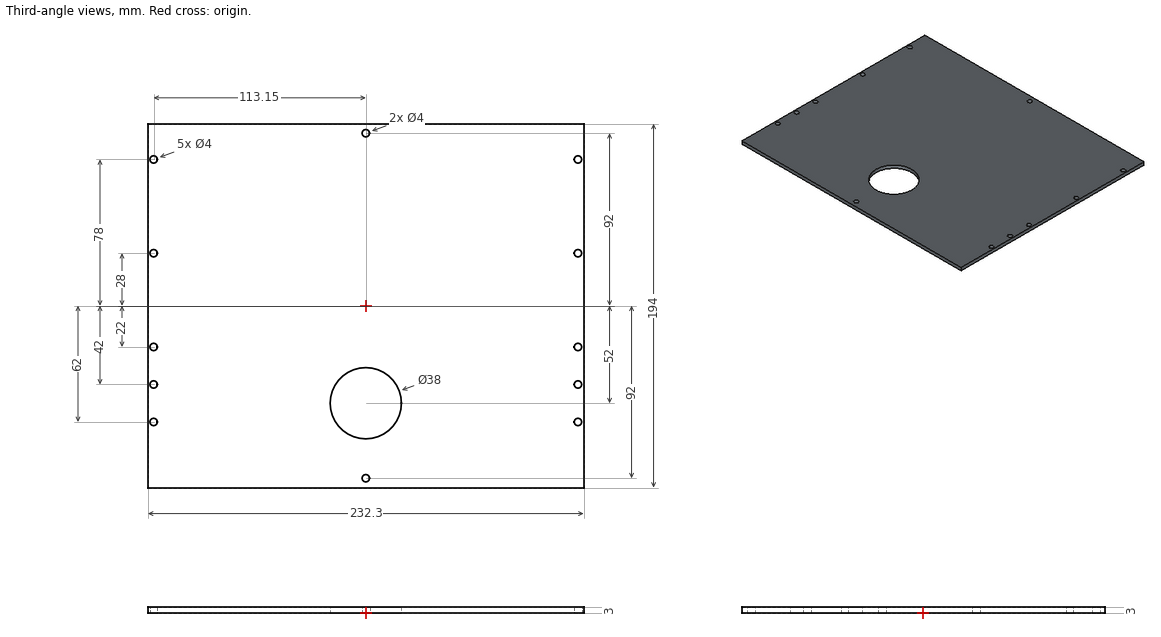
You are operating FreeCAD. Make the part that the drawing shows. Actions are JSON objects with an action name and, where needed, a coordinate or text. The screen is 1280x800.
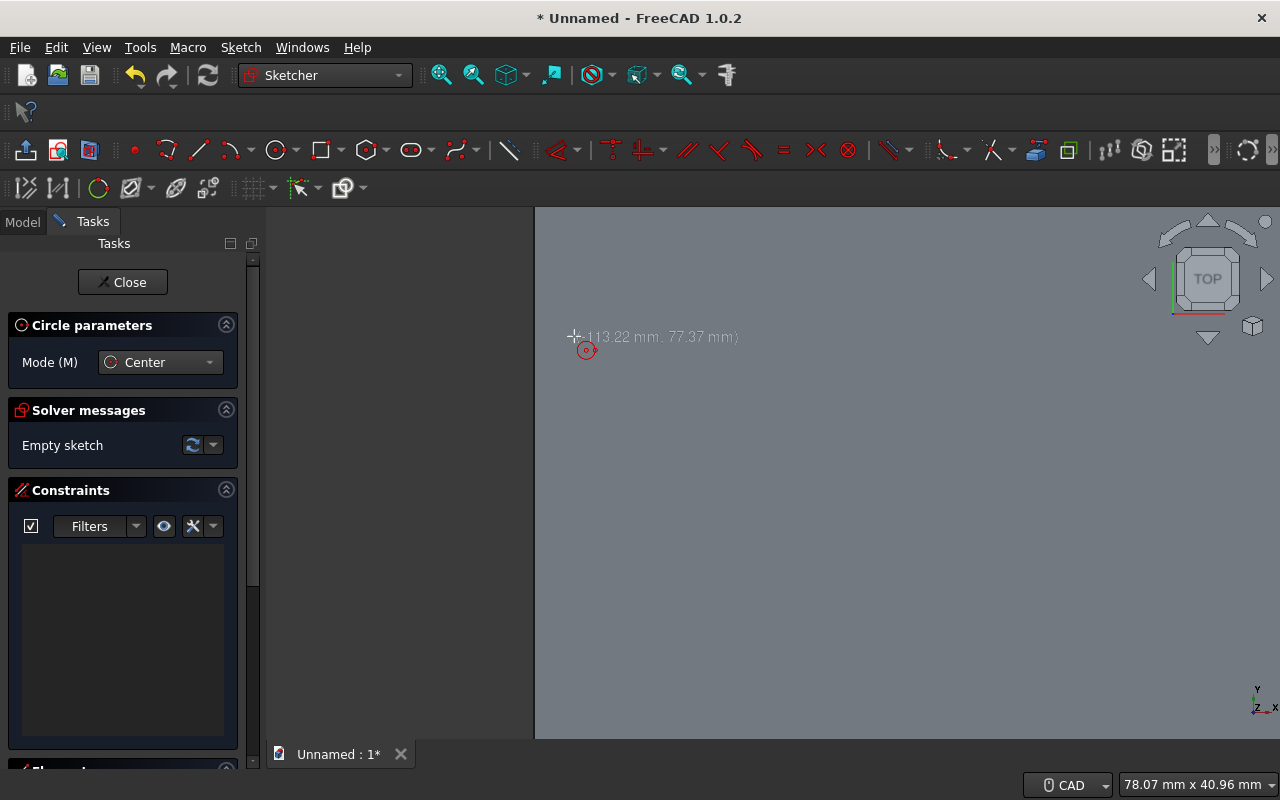
{"action": "scroll", "coordinate": [588, 321], "scroll_direction": "down", "scroll_amount": 9}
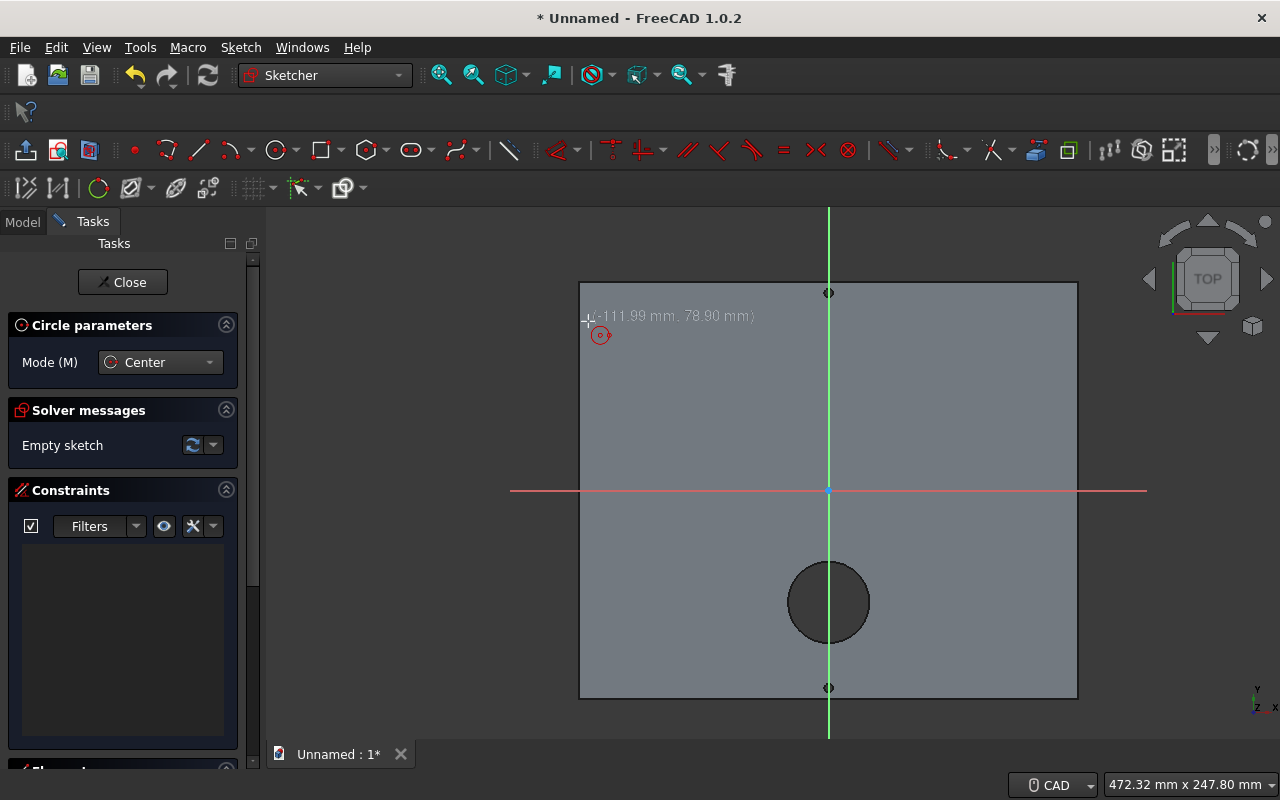
{"action": "left_click", "coordinate": [586, 323]}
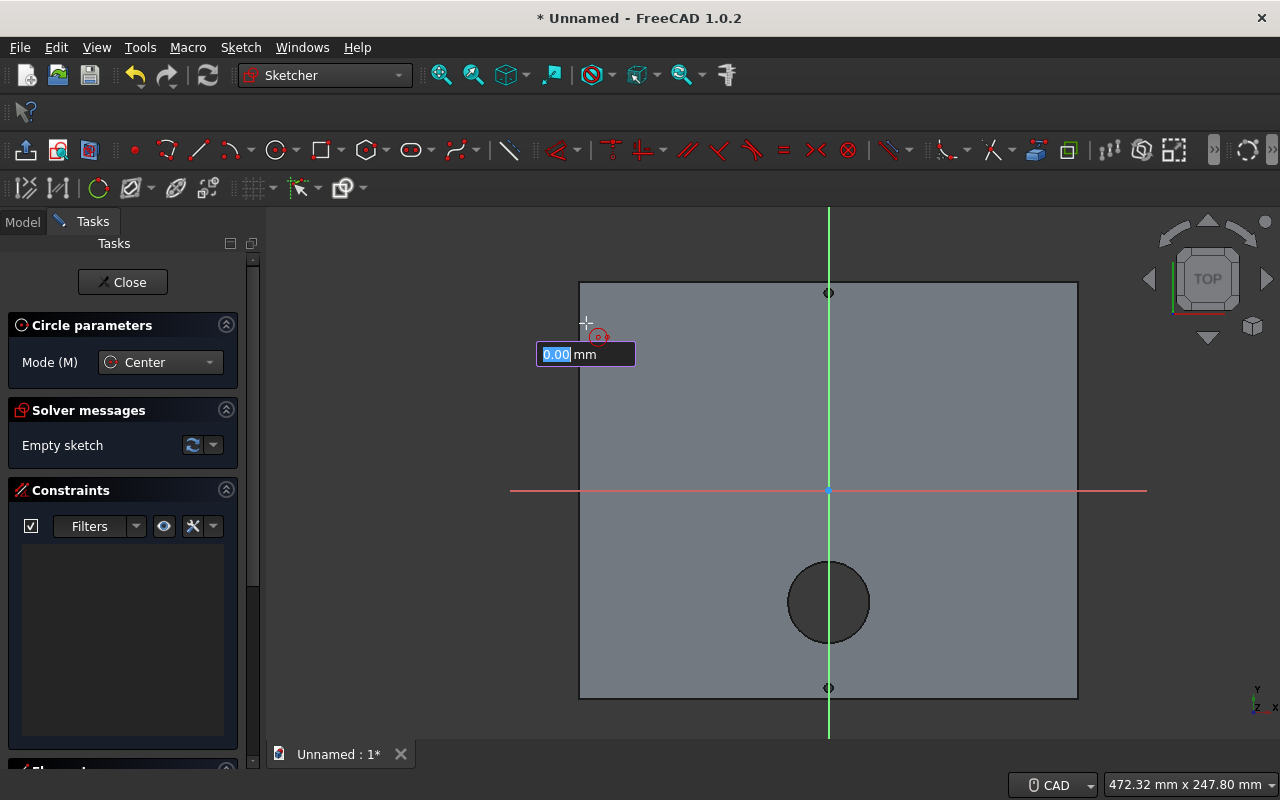
{"action": "scroll", "coordinate": [589, 320], "scroll_direction": "up", "scroll_amount": 7}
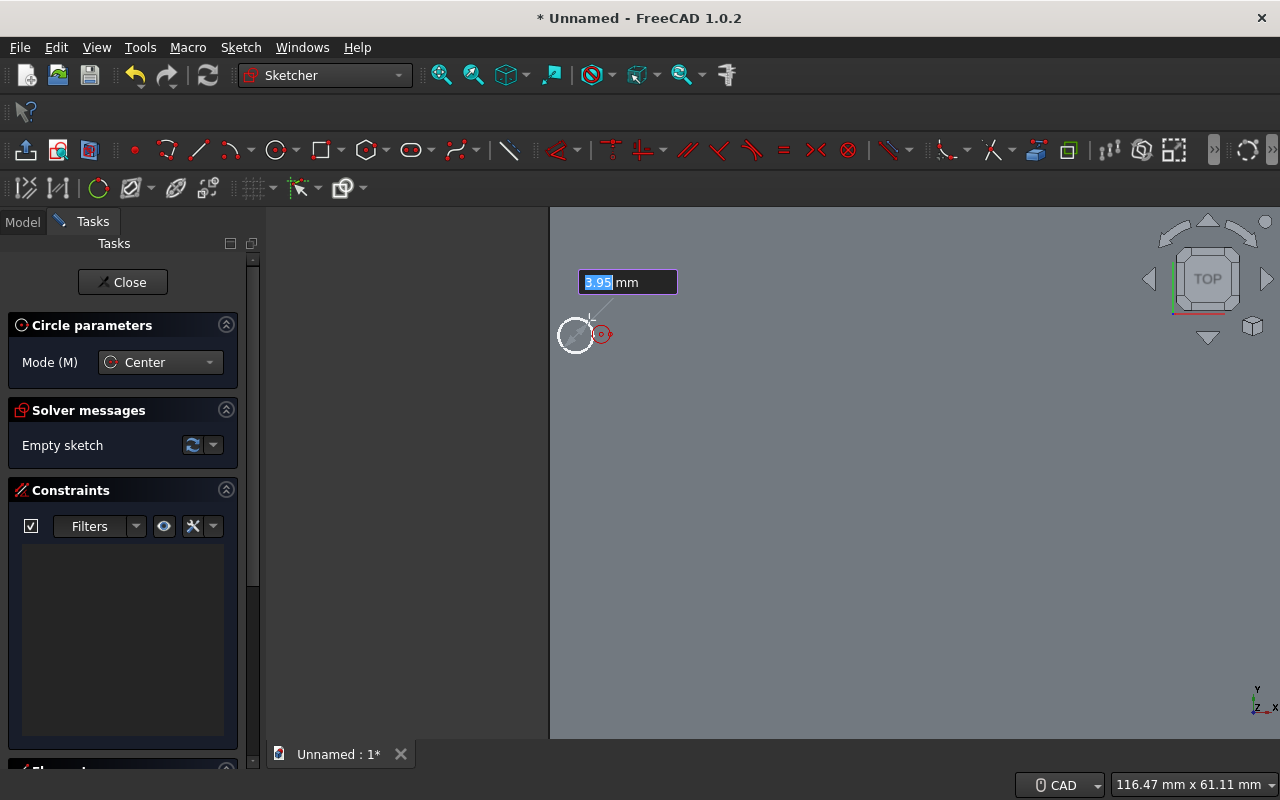
{"action": "left_click", "coordinate": [587, 320]}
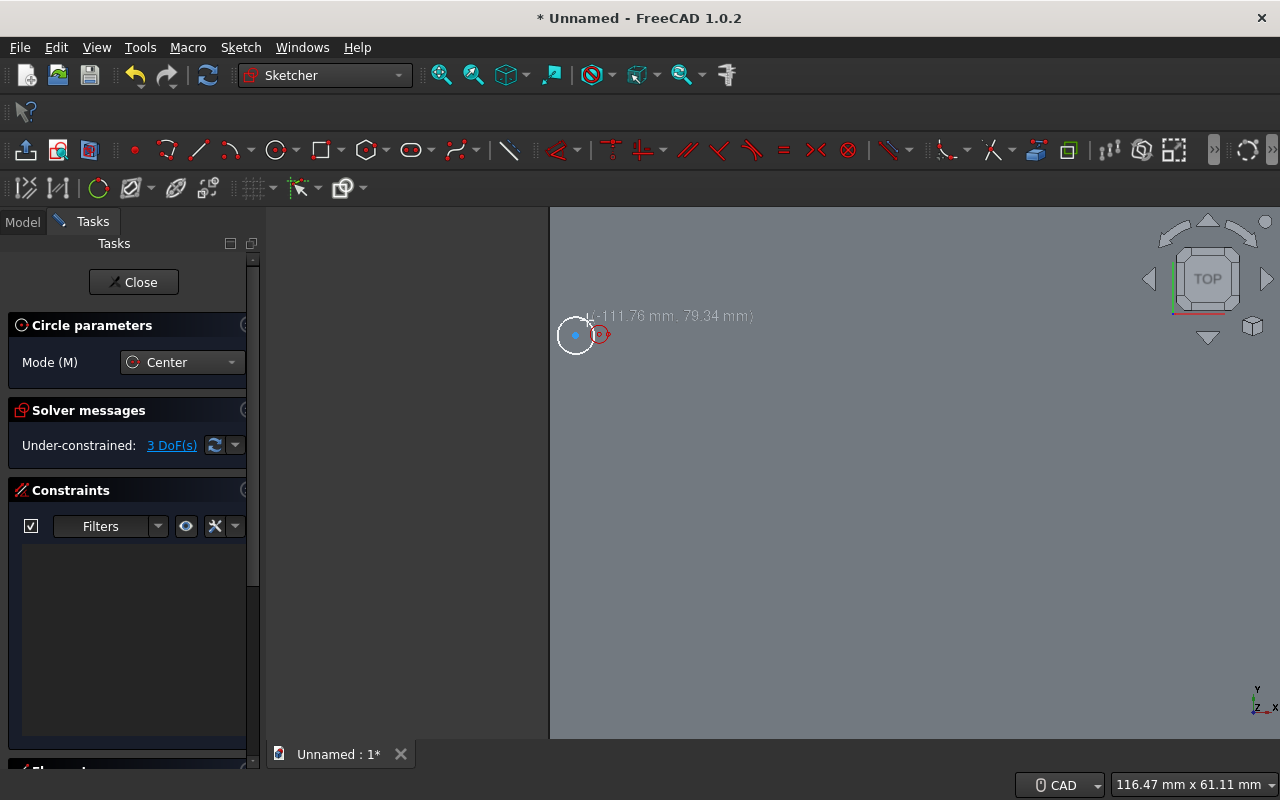
{"action": "scroll", "coordinate": [589, 319], "scroll_direction": "down", "scroll_amount": 7}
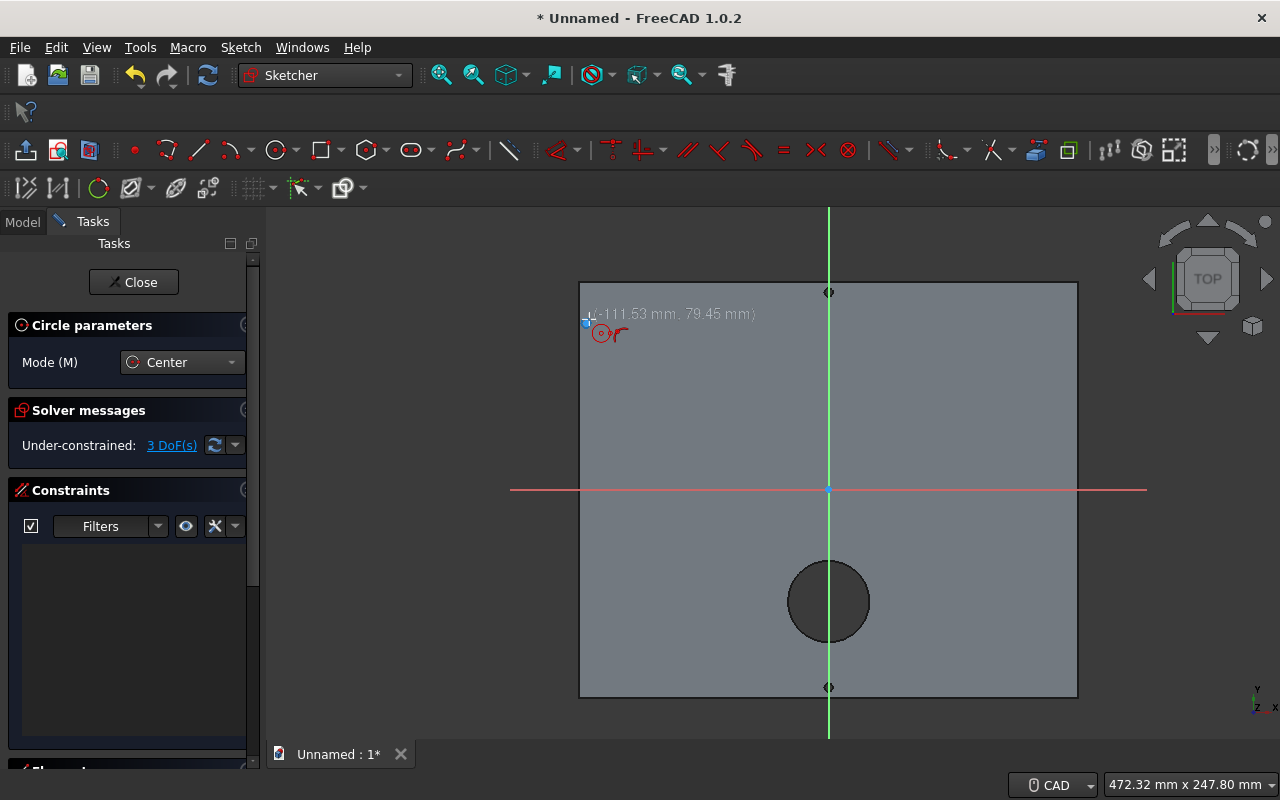
{"action": "scroll", "coordinate": [586, 430], "scroll_direction": "up", "scroll_amount": 9}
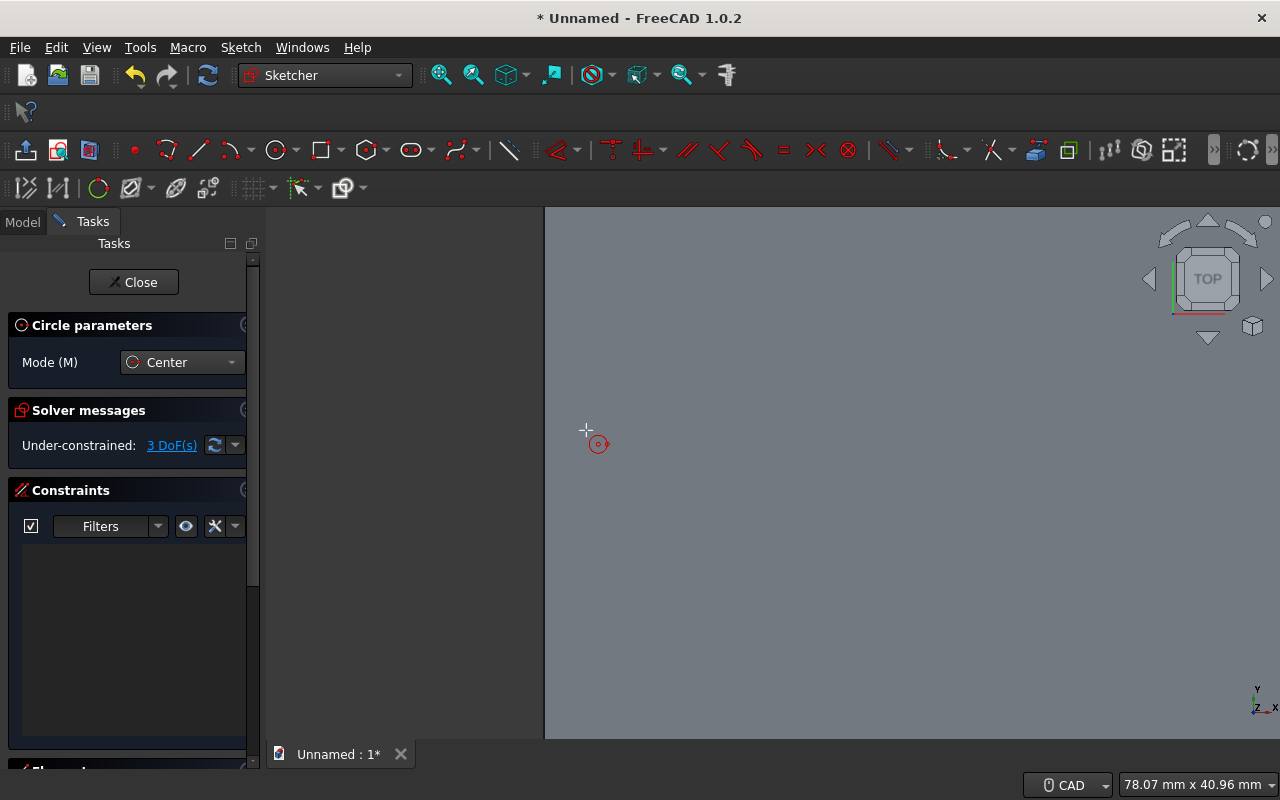
{"action": "scroll", "coordinate": [586, 431], "scroll_direction": "down", "scroll_amount": 9}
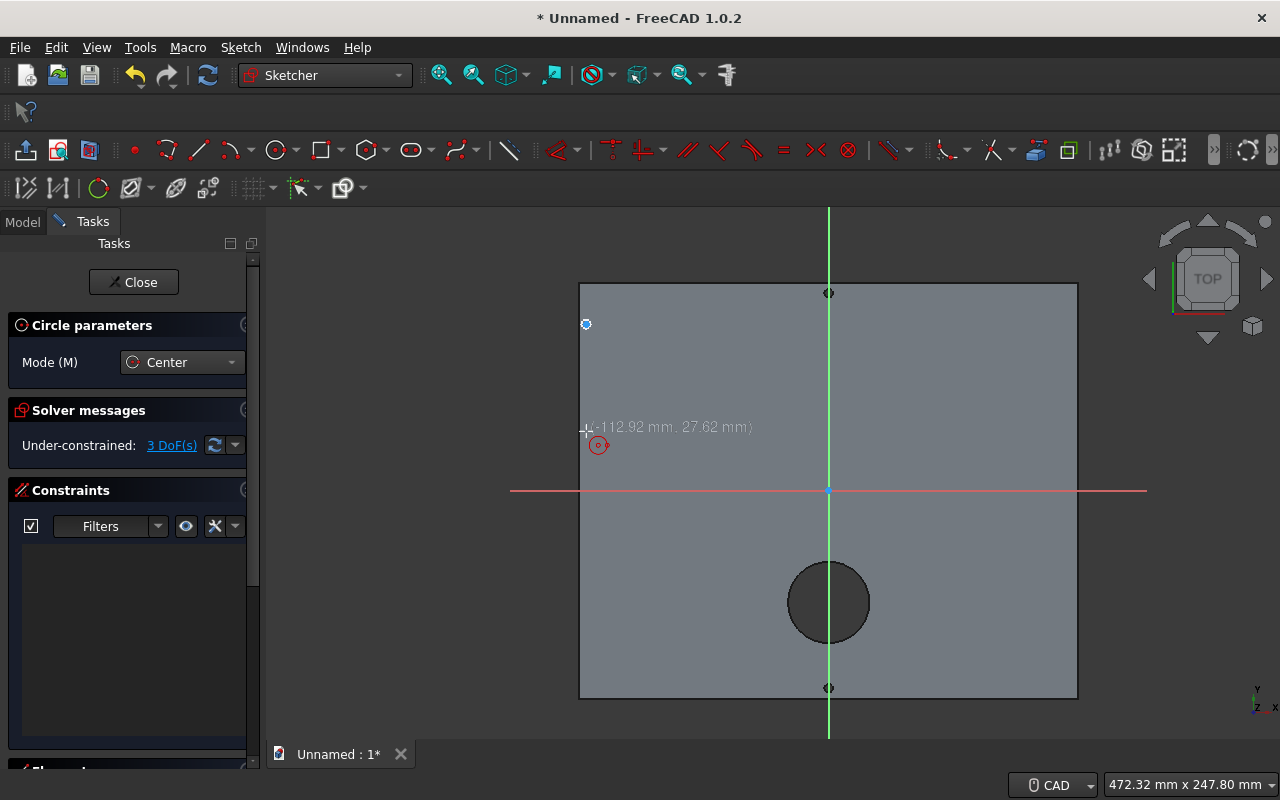
{"action": "left_click", "coordinate": [586, 431]}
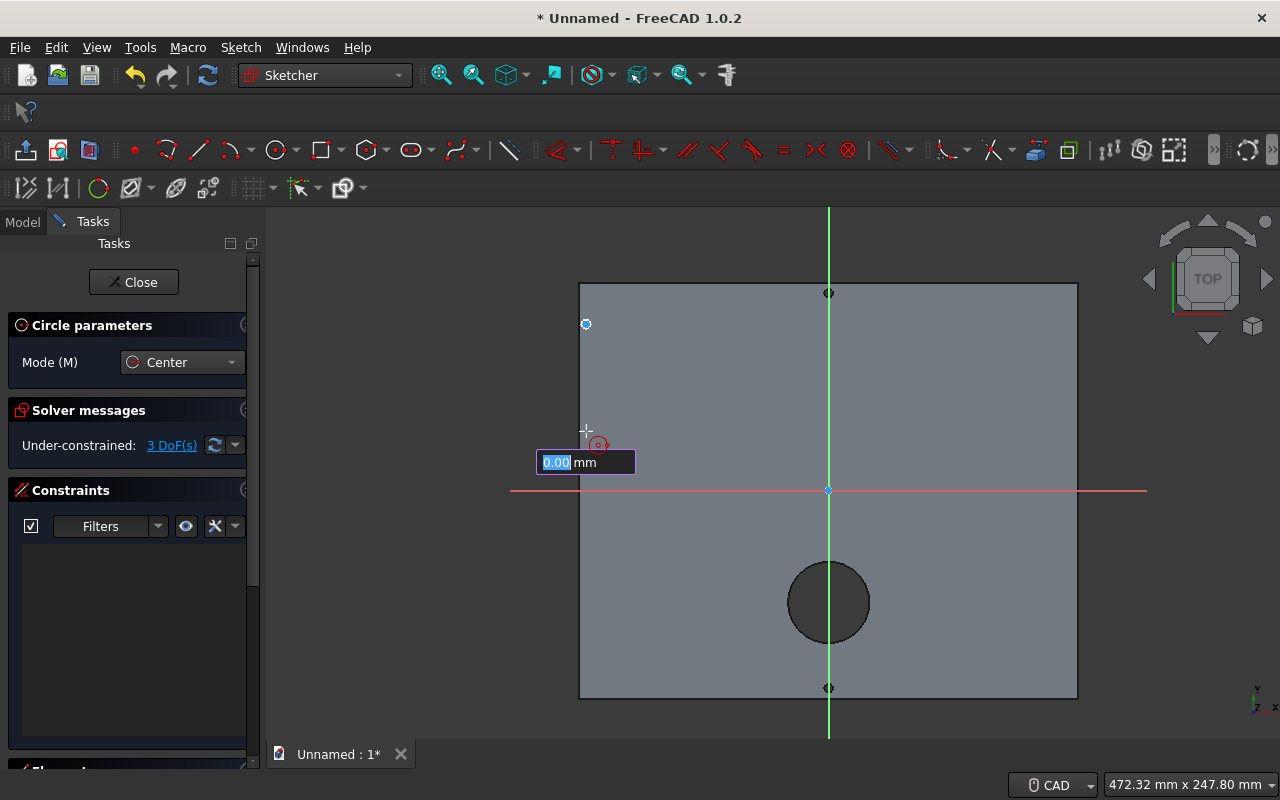
{"action": "scroll", "coordinate": [589, 428], "scroll_direction": "up", "scroll_amount": 7}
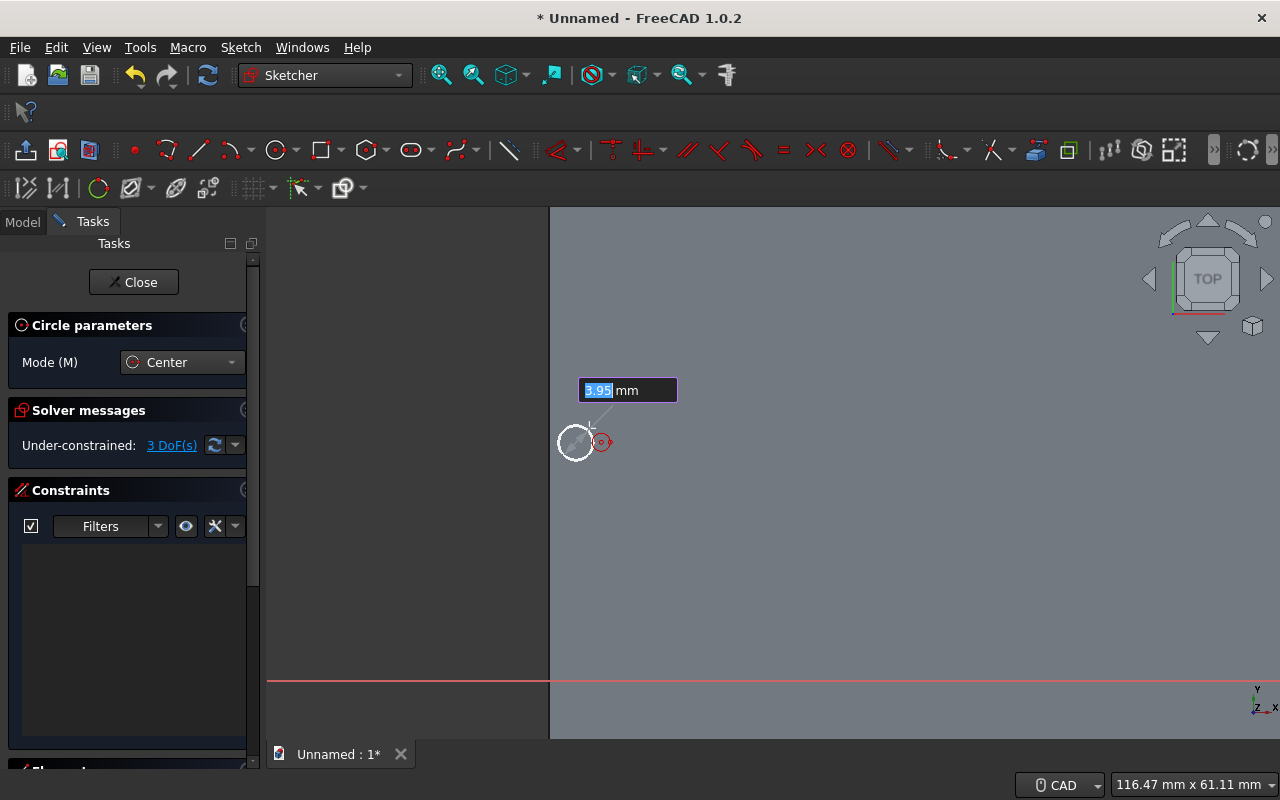
{"action": "left_click", "coordinate": [587, 425]}